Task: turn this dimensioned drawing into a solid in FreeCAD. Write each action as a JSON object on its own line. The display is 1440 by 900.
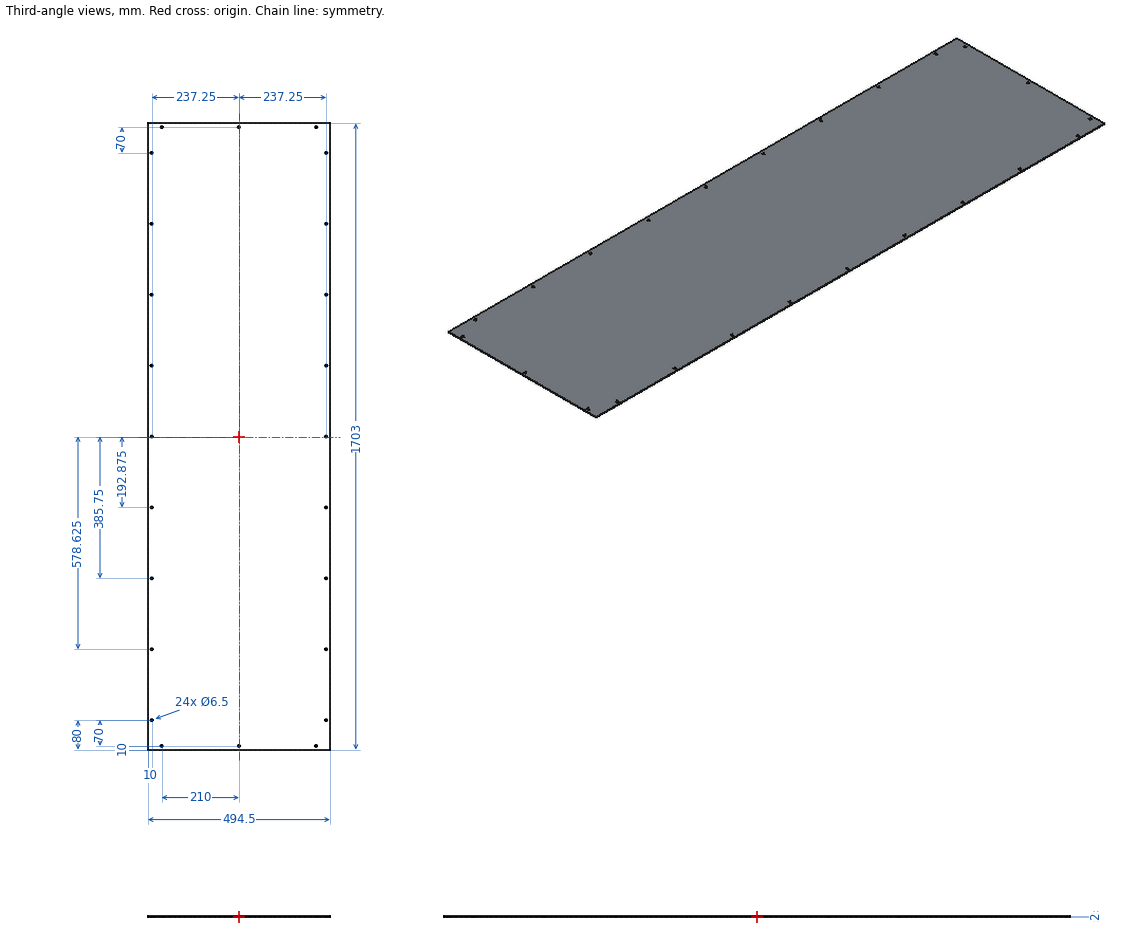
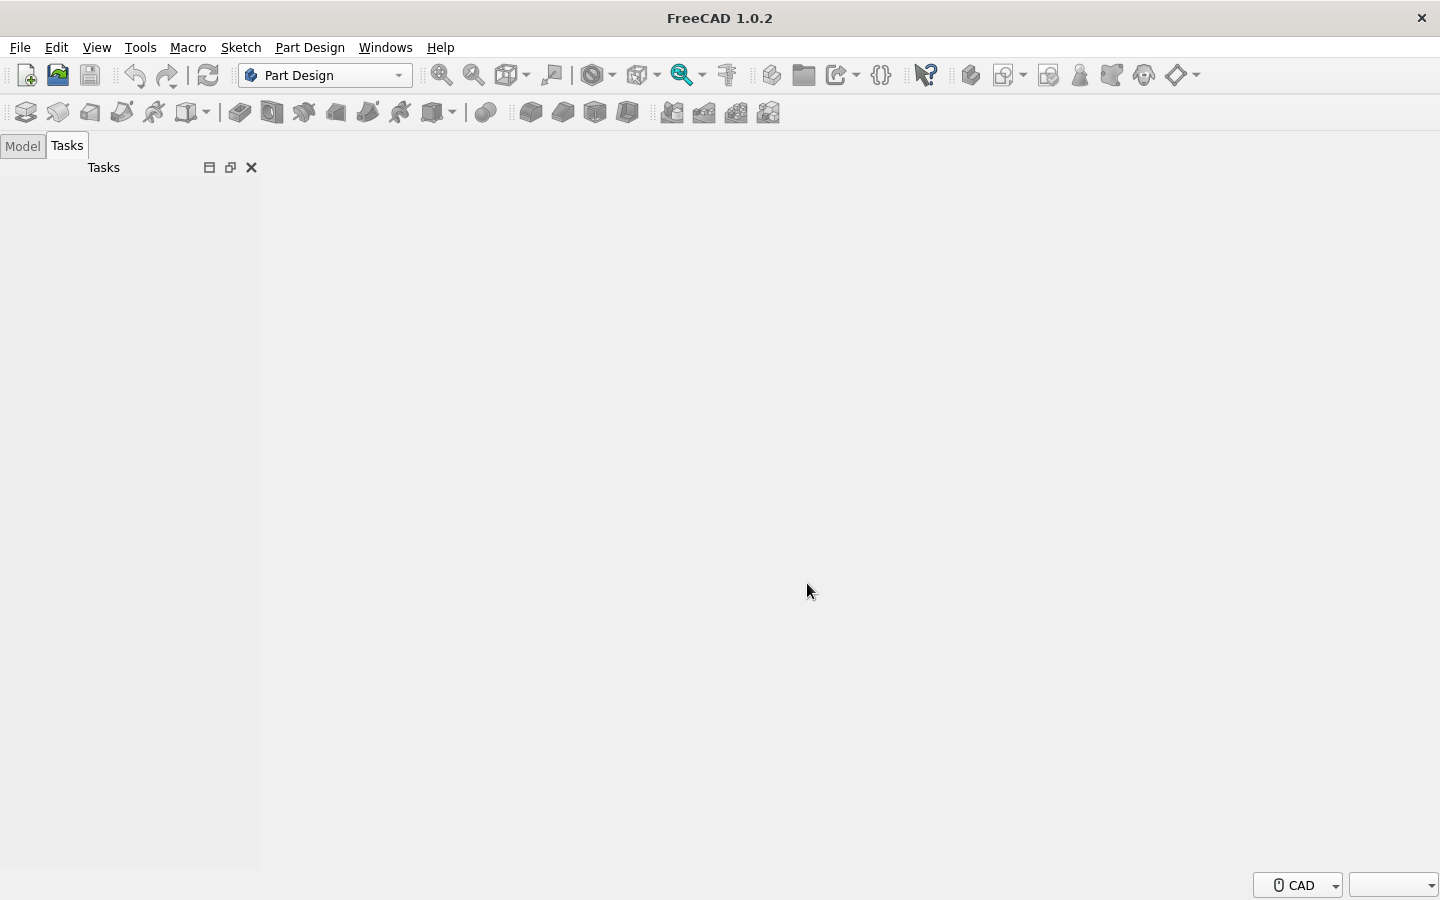
{"action": "left_click", "coordinate": [26, 76]}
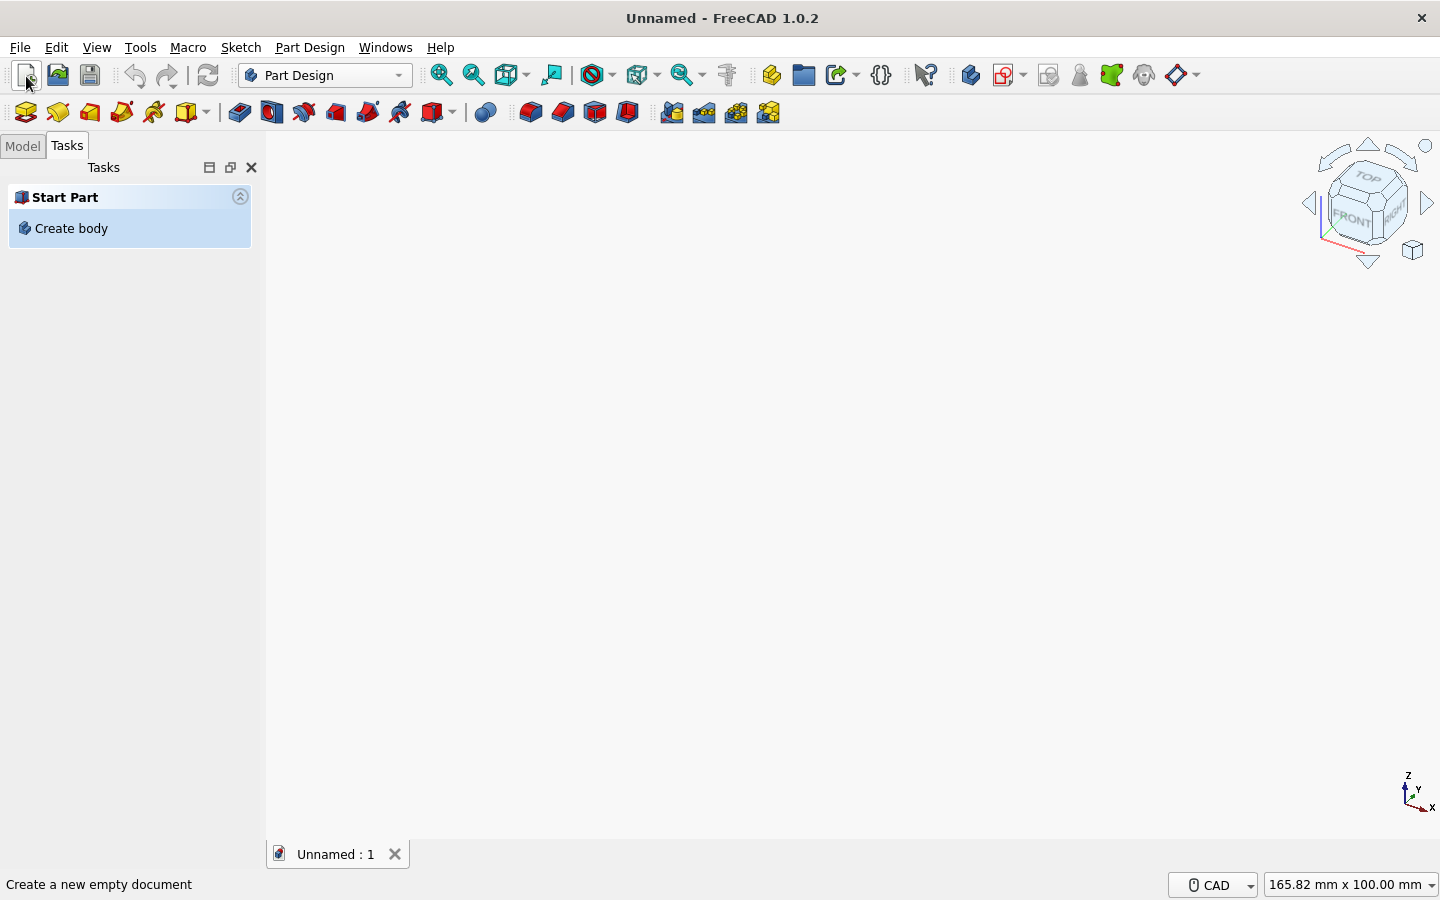
{"action": "left_click", "coordinate": [1004, 76]}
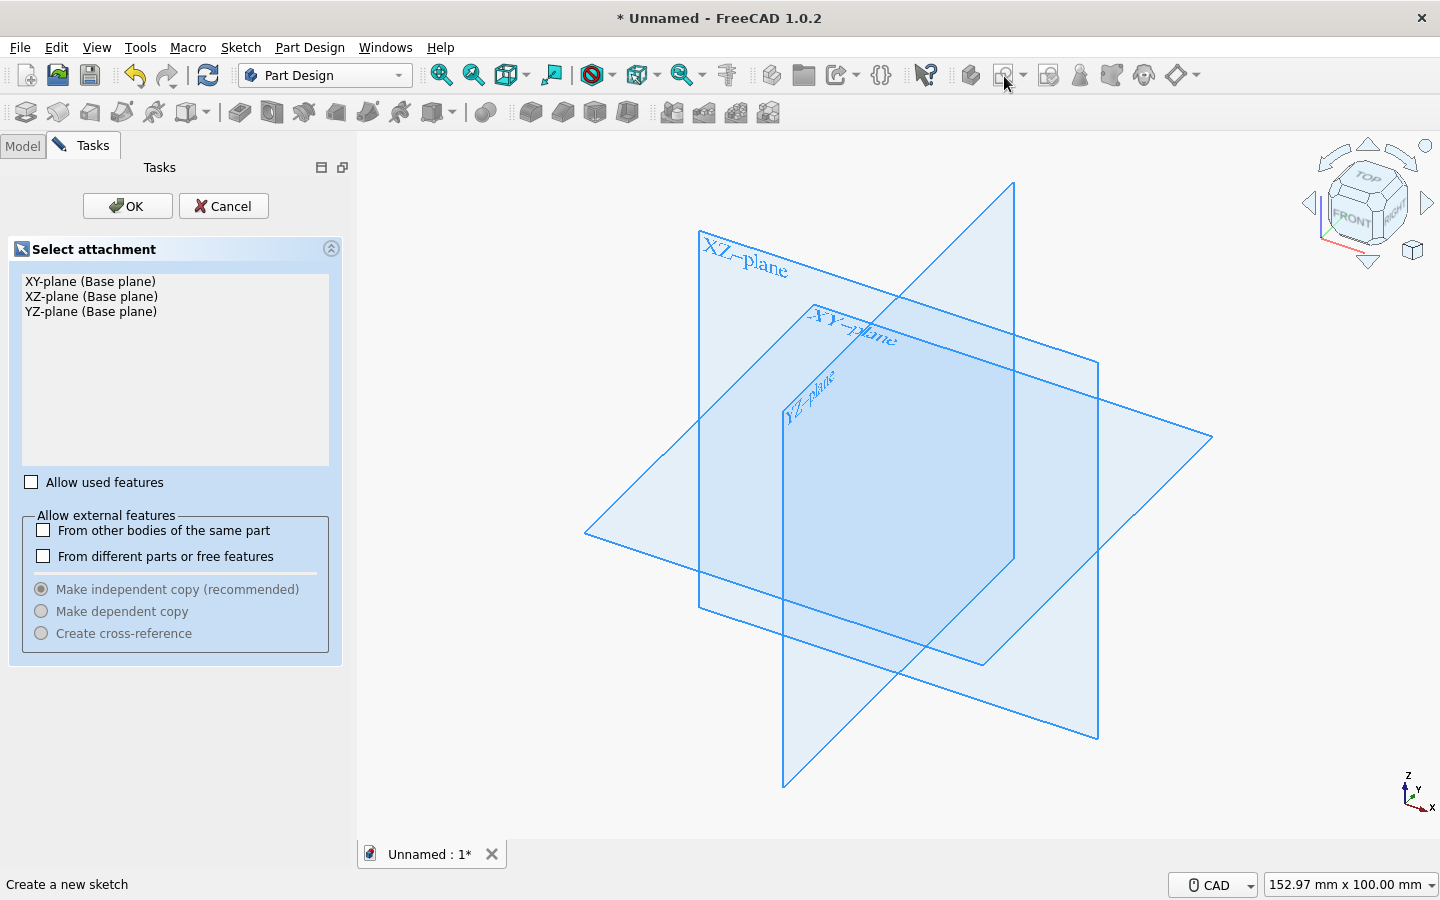
{"action": "left_click", "coordinate": [82, 282]}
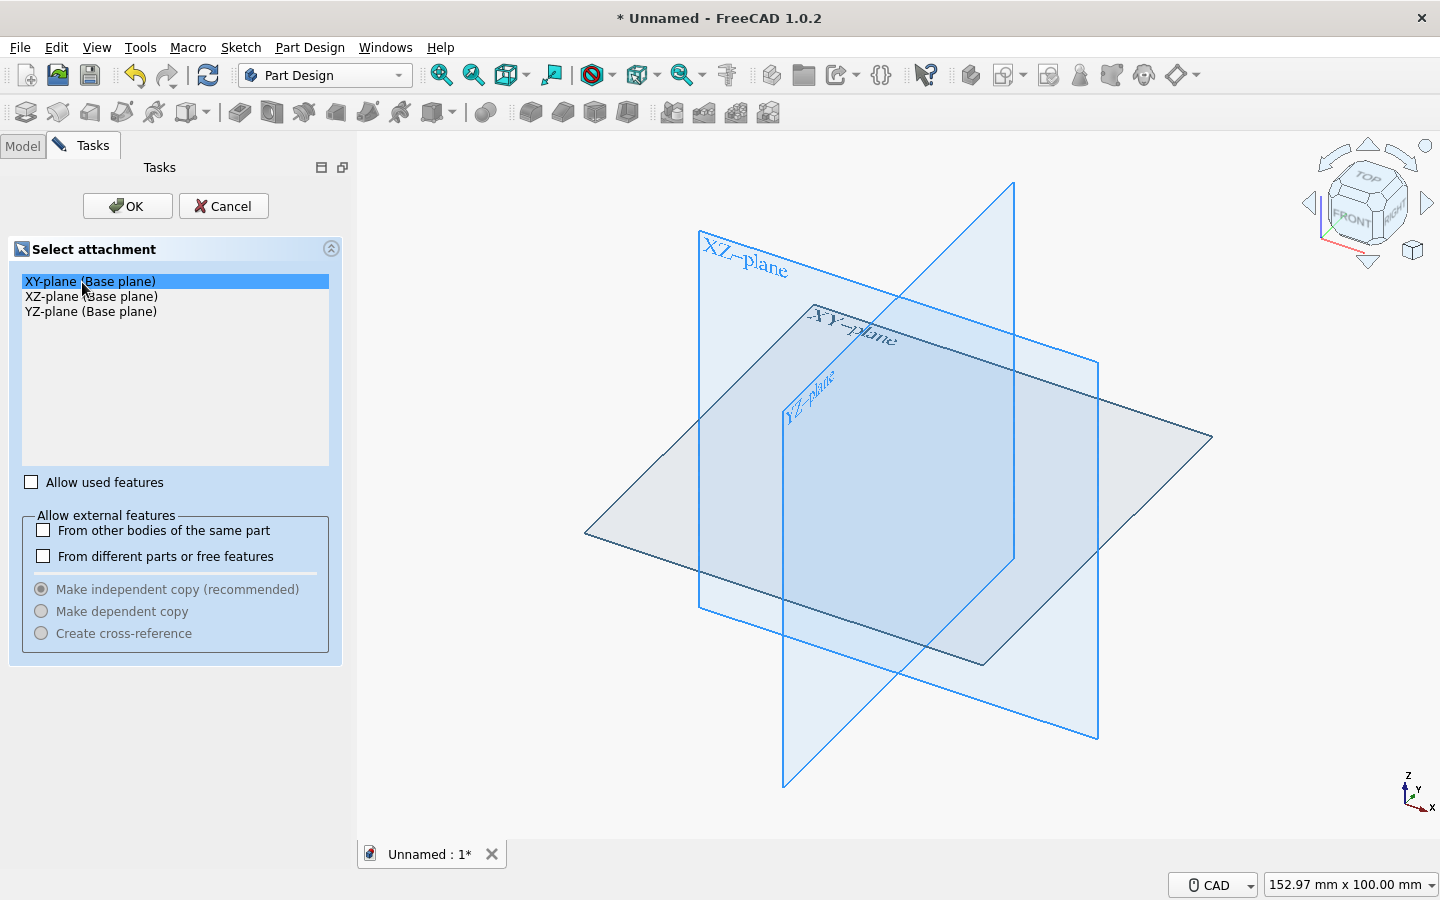
{"action": "left_click", "coordinate": [128, 206]}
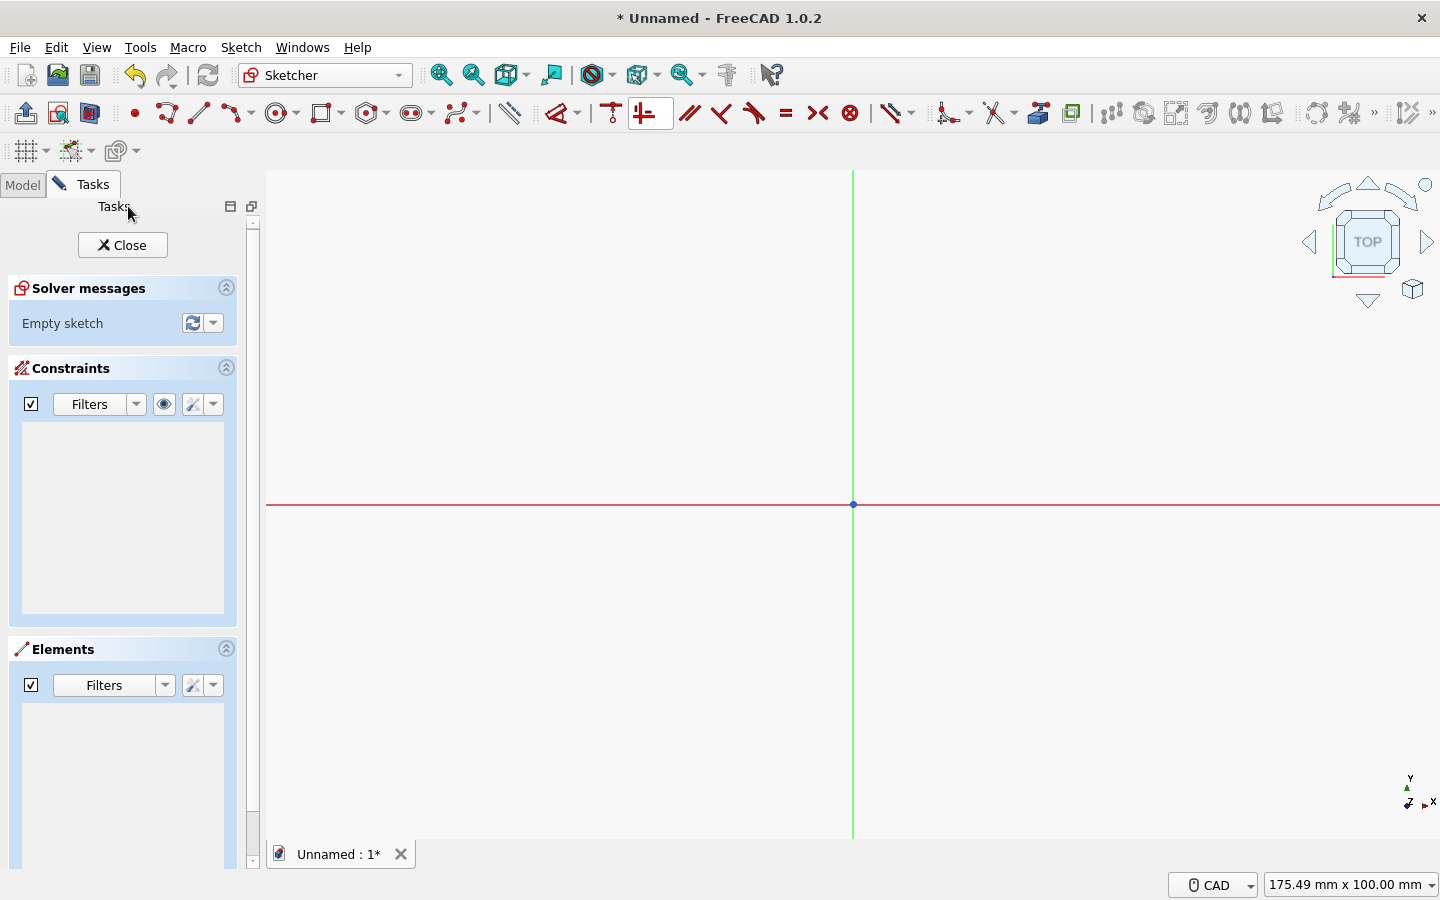
{"action": "scroll", "coordinate": [782, 504], "scroll_direction": "down", "scroll_amount": 16}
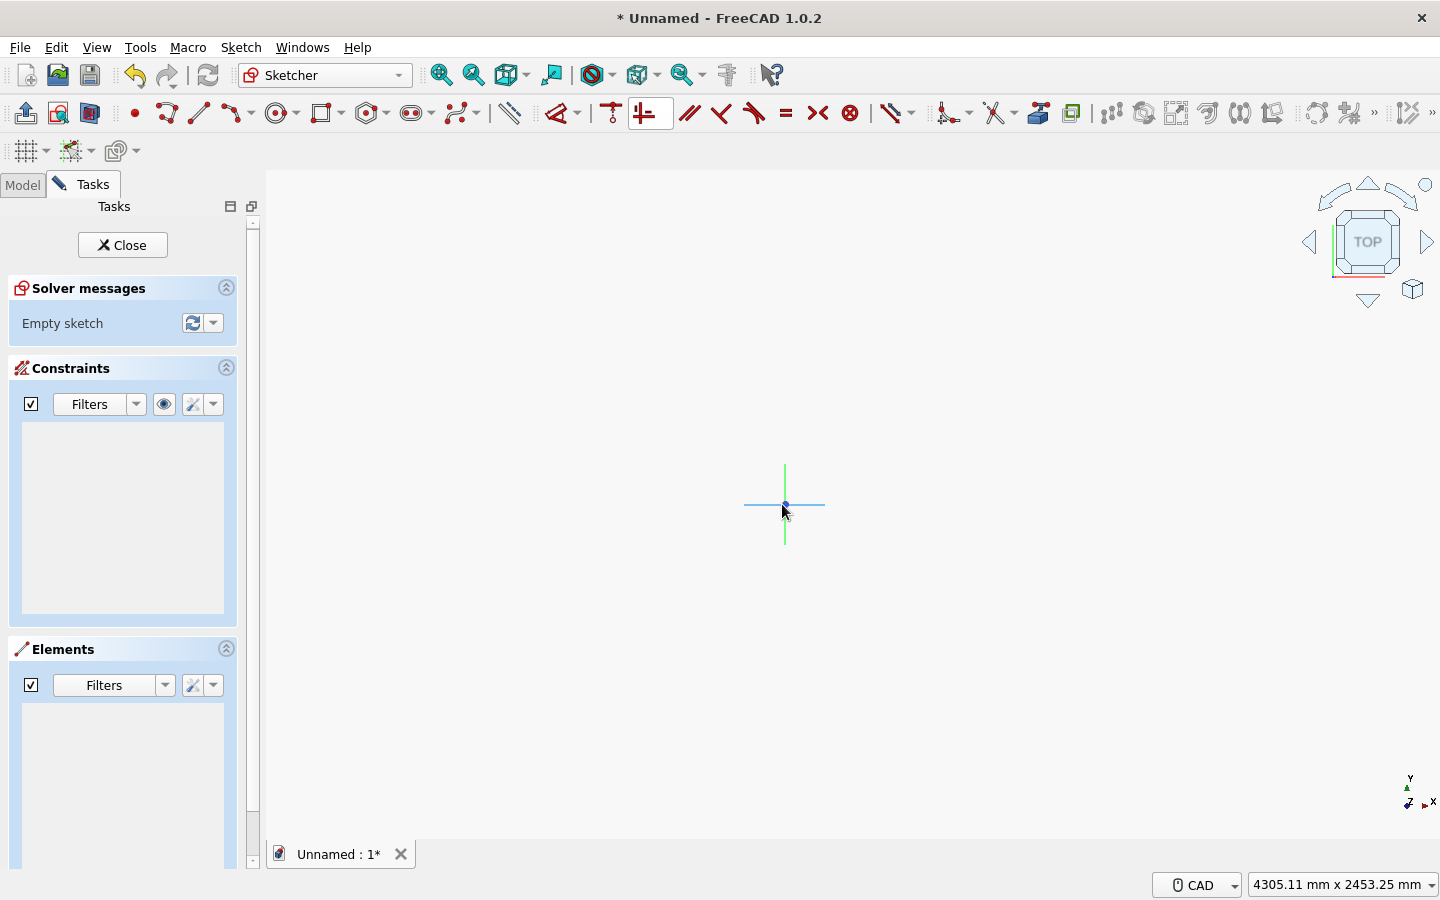
{"action": "key", "text": "g v"}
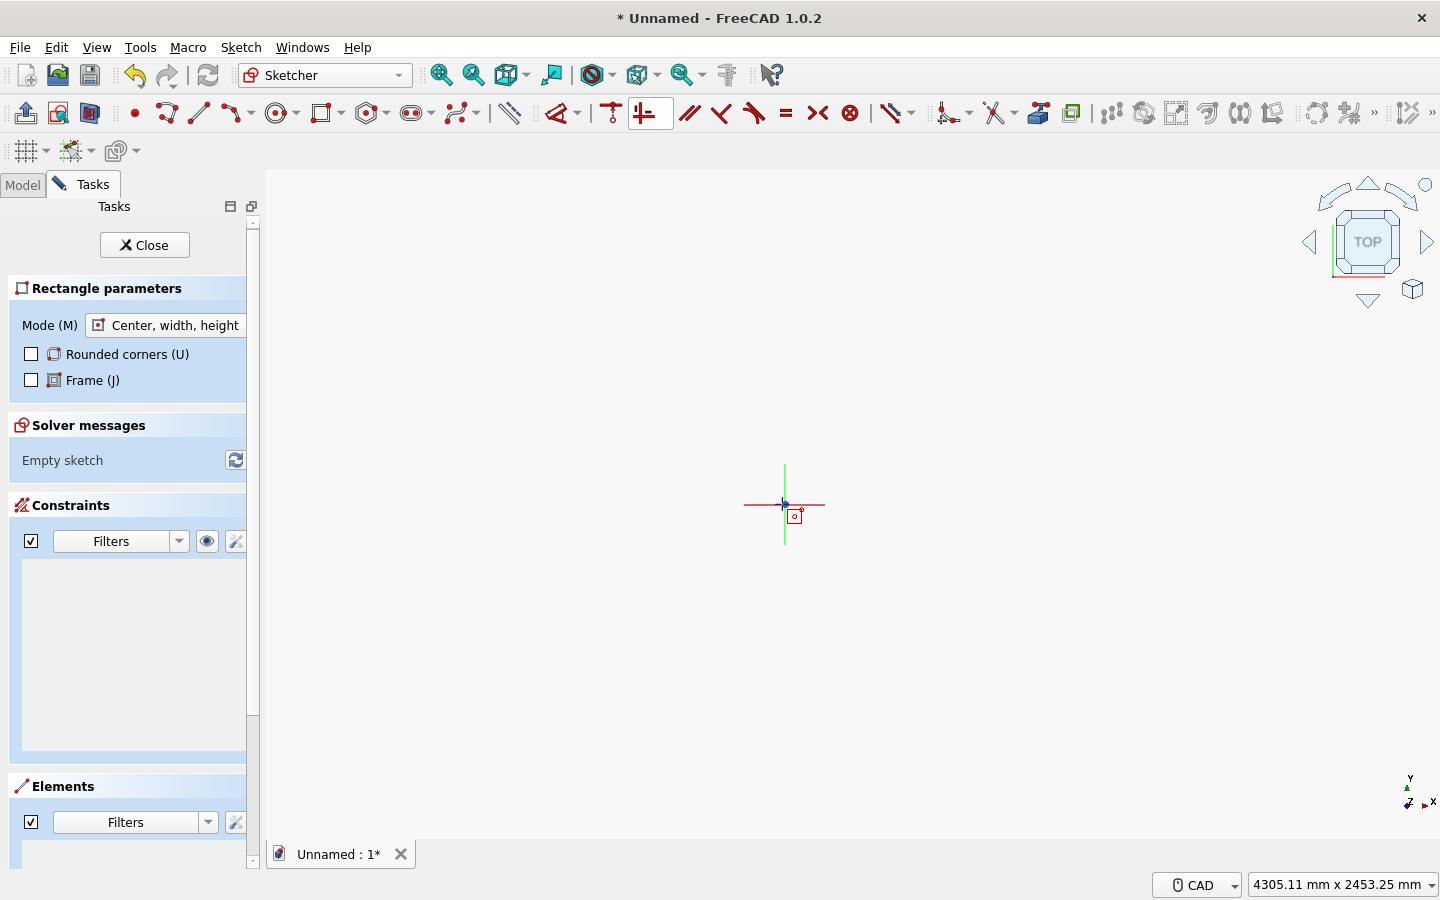
{"action": "left_click", "coordinate": [785, 504]}
{"action": "mouse_move", "coordinate": [853, 272]}